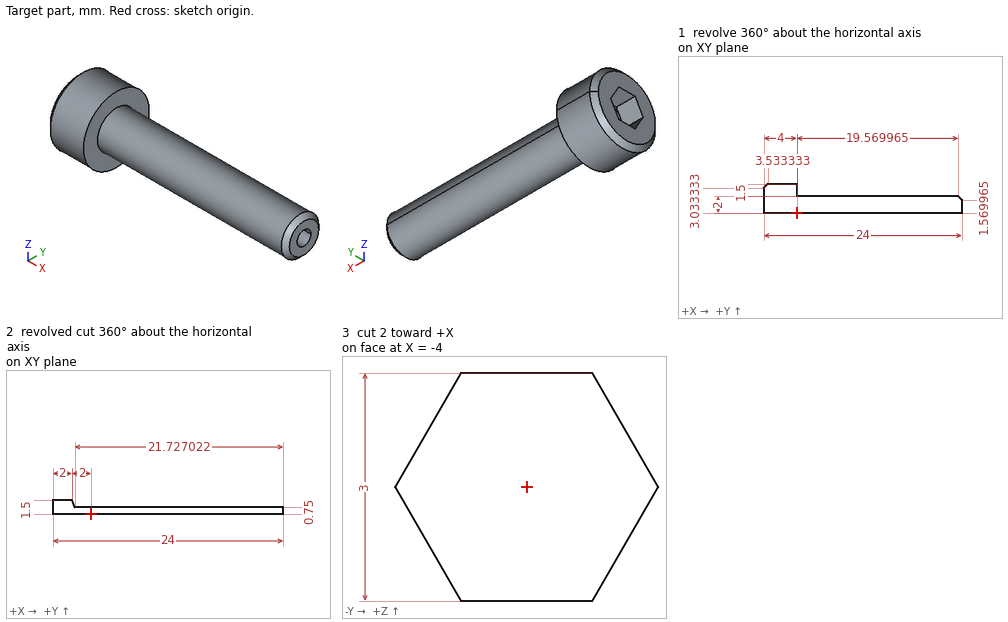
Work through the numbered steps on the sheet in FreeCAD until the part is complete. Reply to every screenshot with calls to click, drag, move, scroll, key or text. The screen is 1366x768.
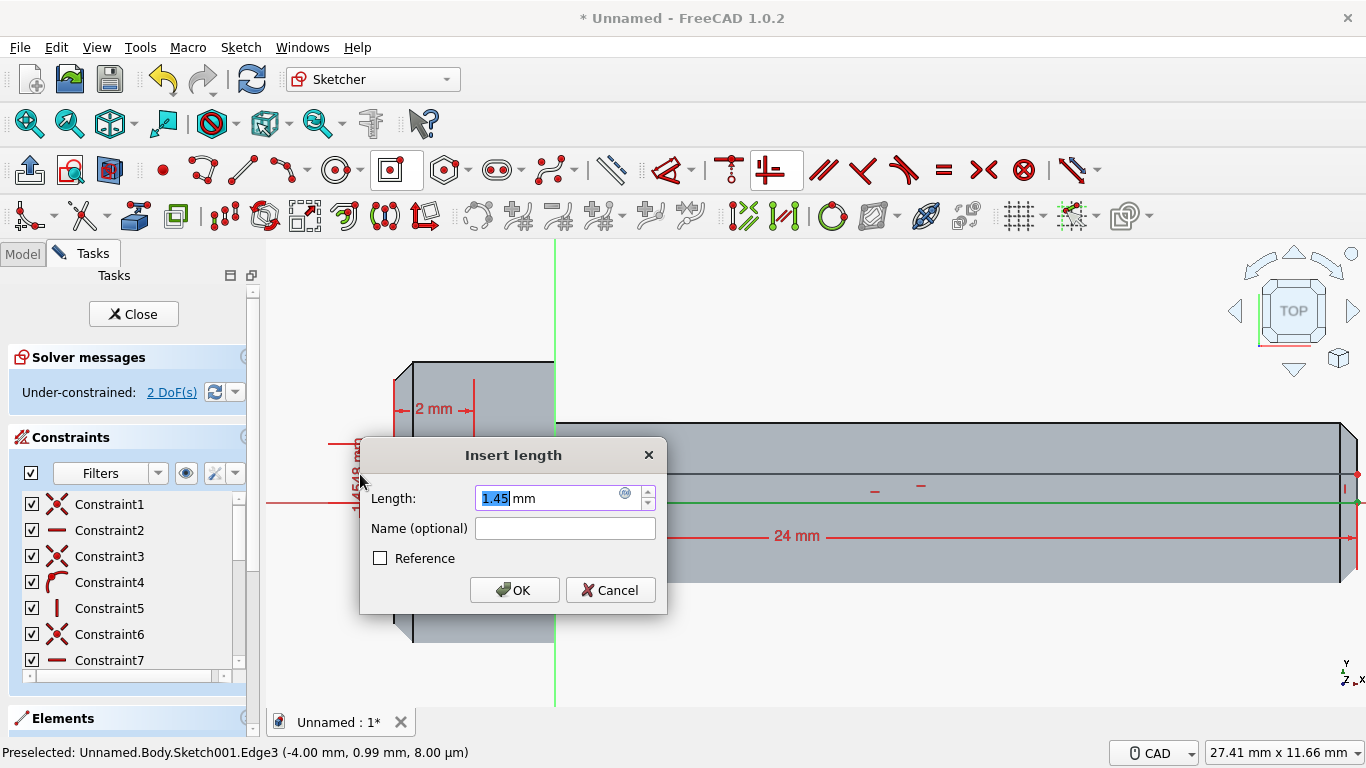
text(1.5)
key(Return)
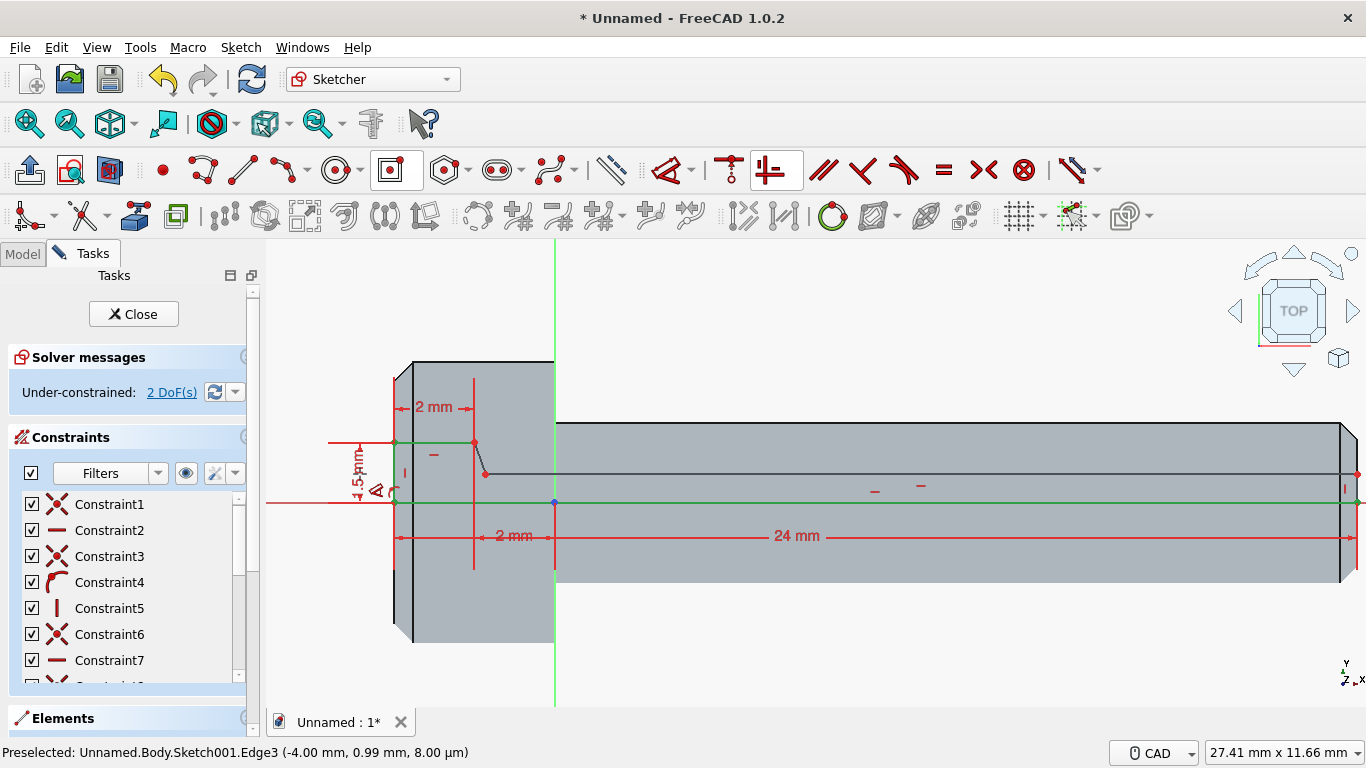
scroll(487, 474, down, 2)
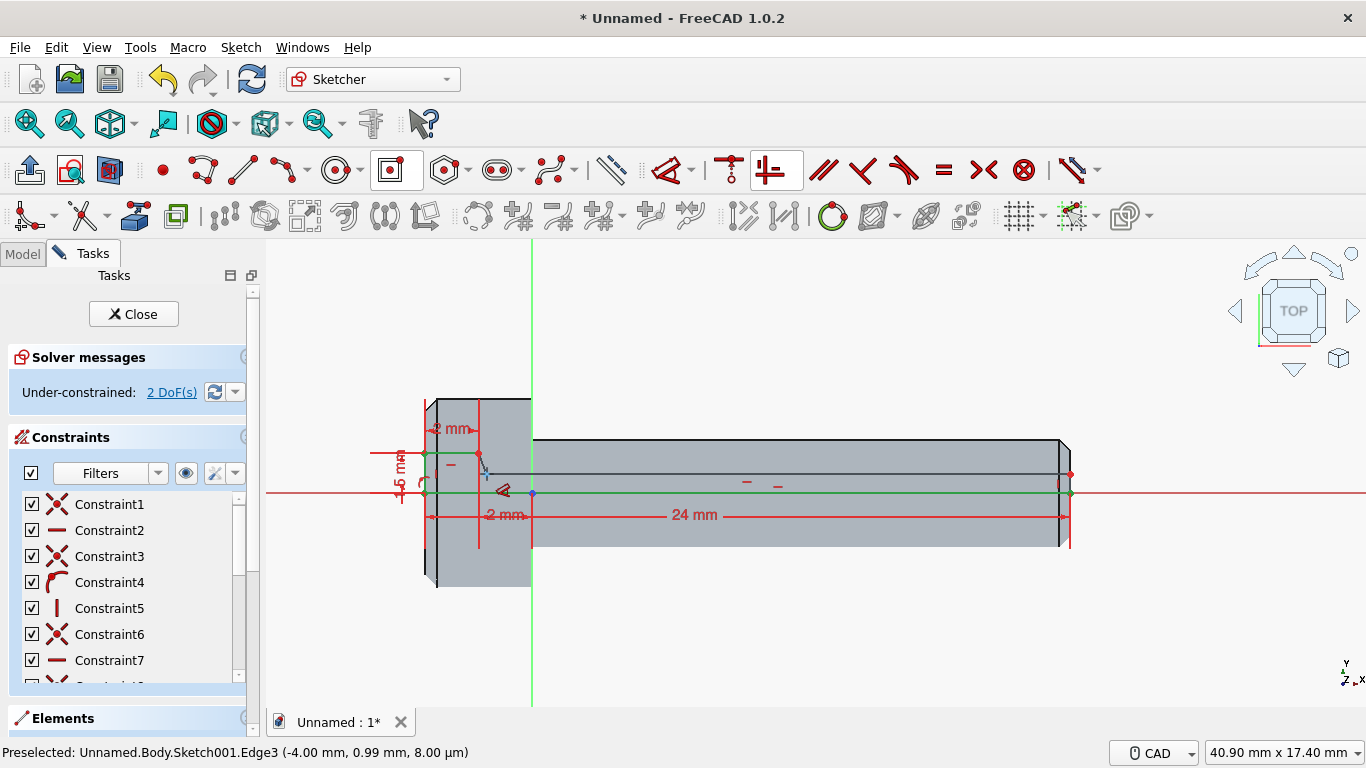
scroll(1070, 486, up, 4)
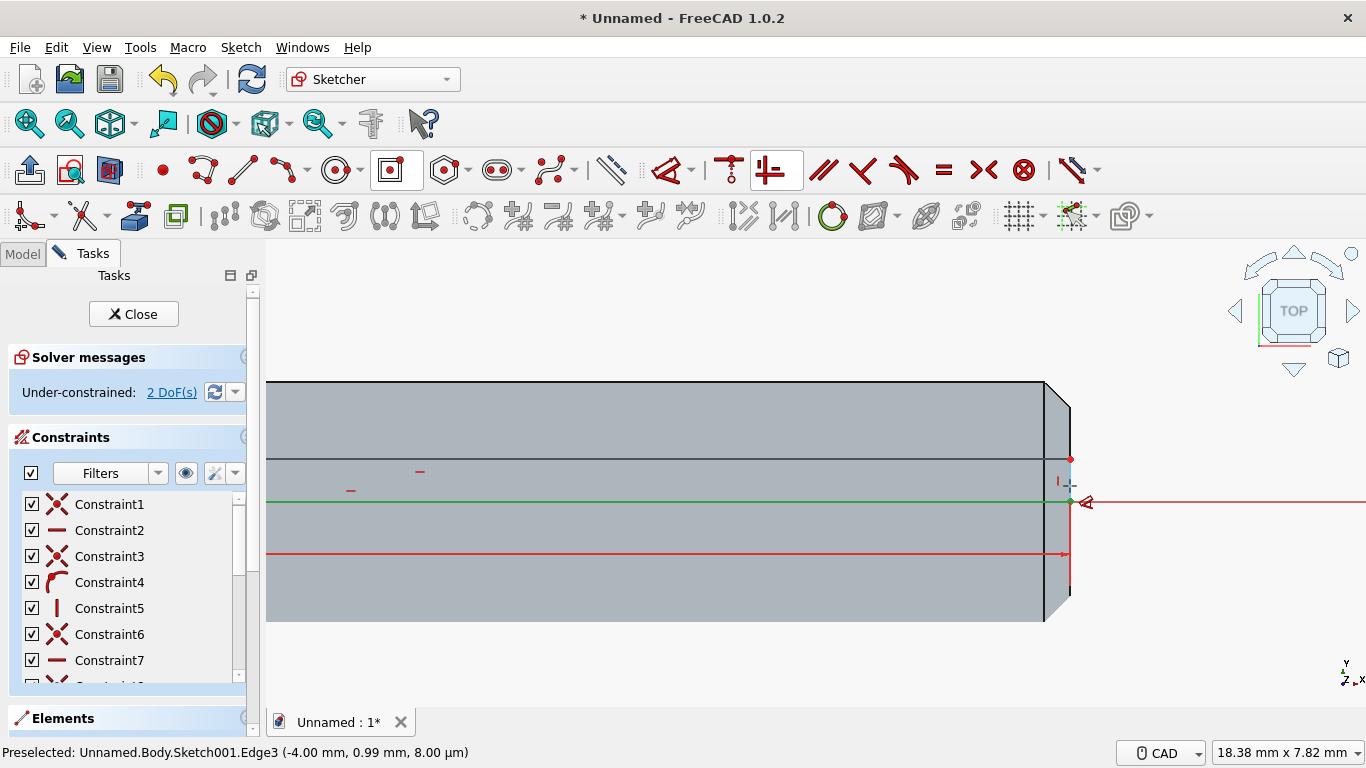
click(1070, 485)
click(1104, 481)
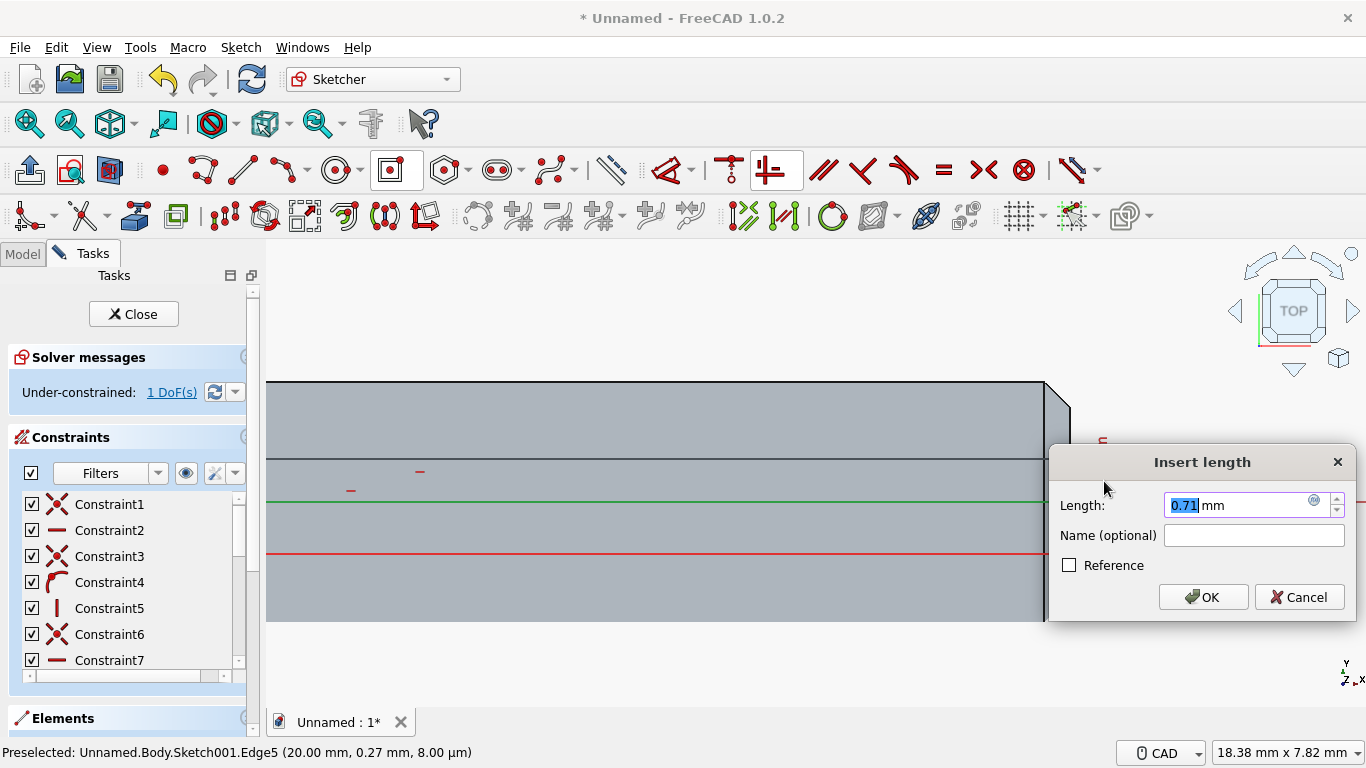
text(0.75)
key(Return)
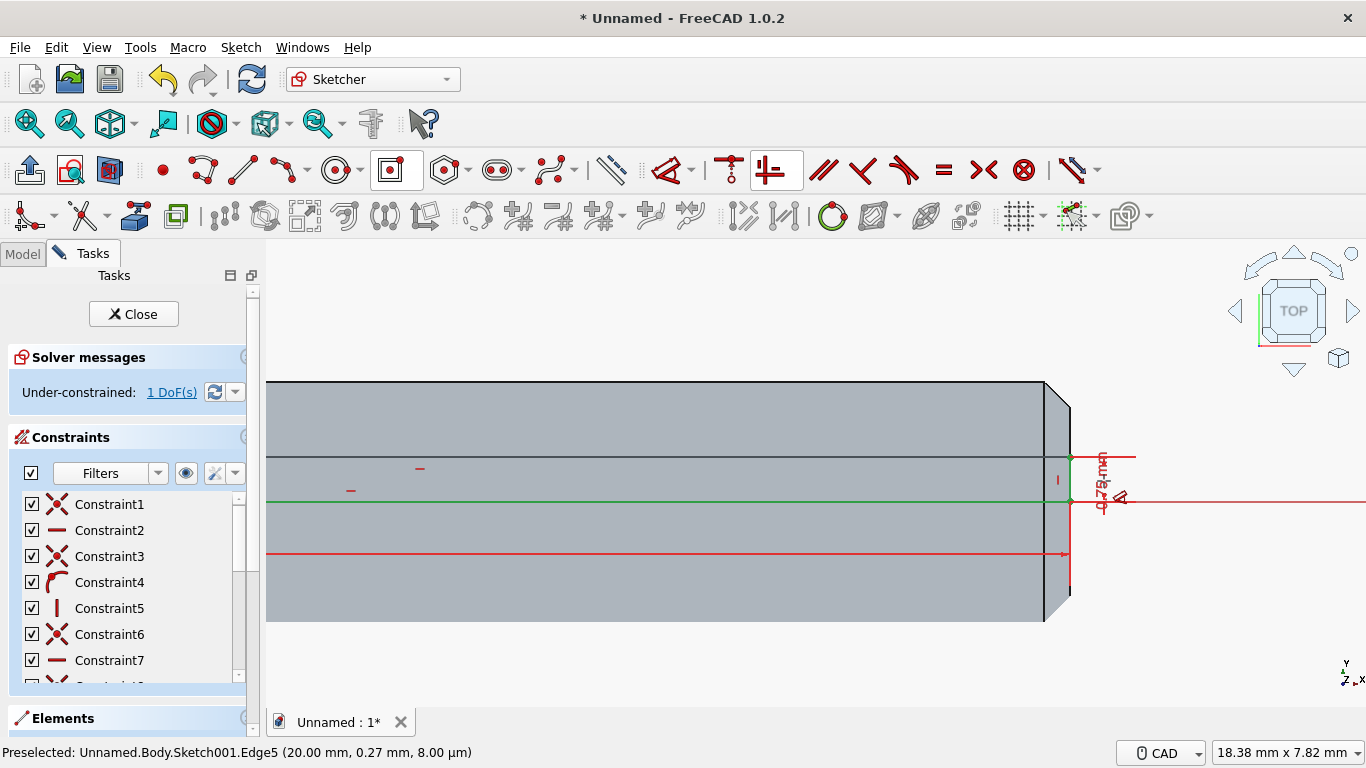
click(680, 457)
click(682, 423)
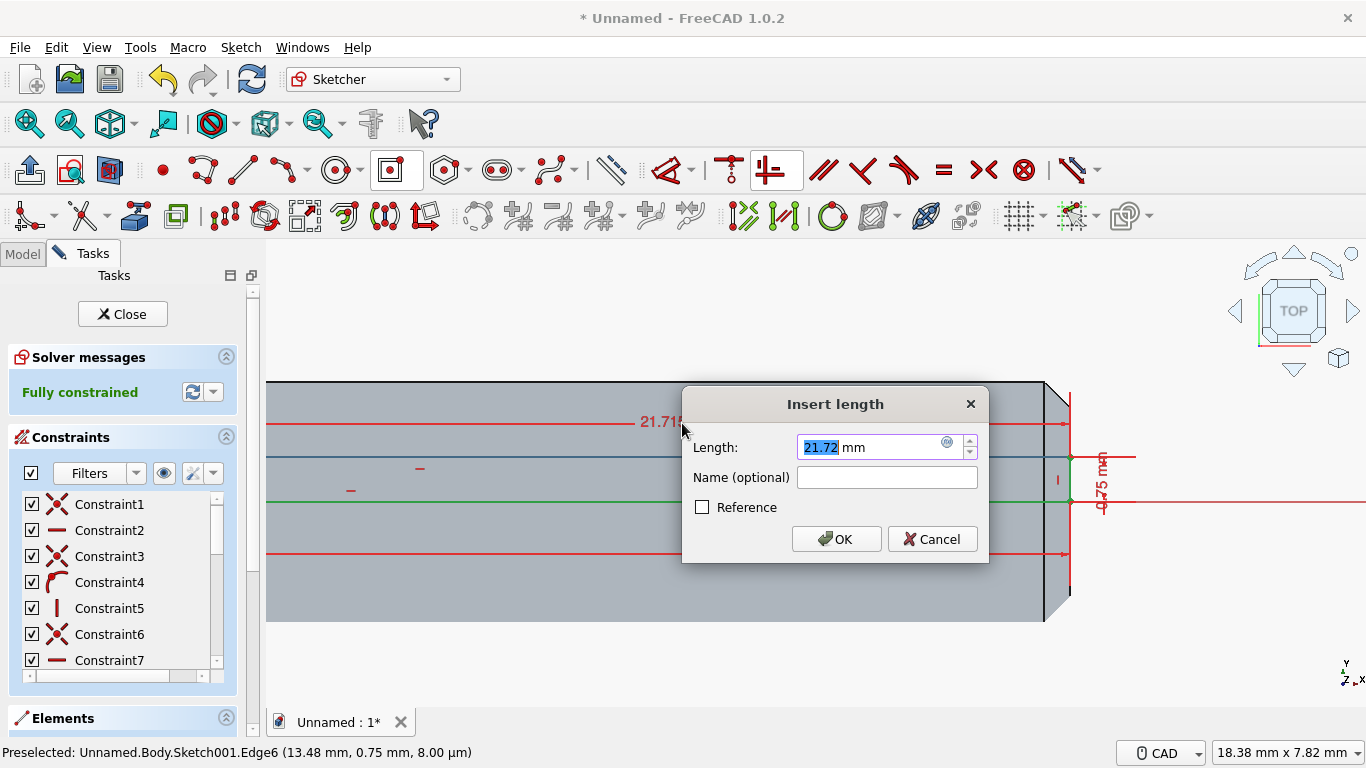
text(21.727022)
key(Return)
key(Escape)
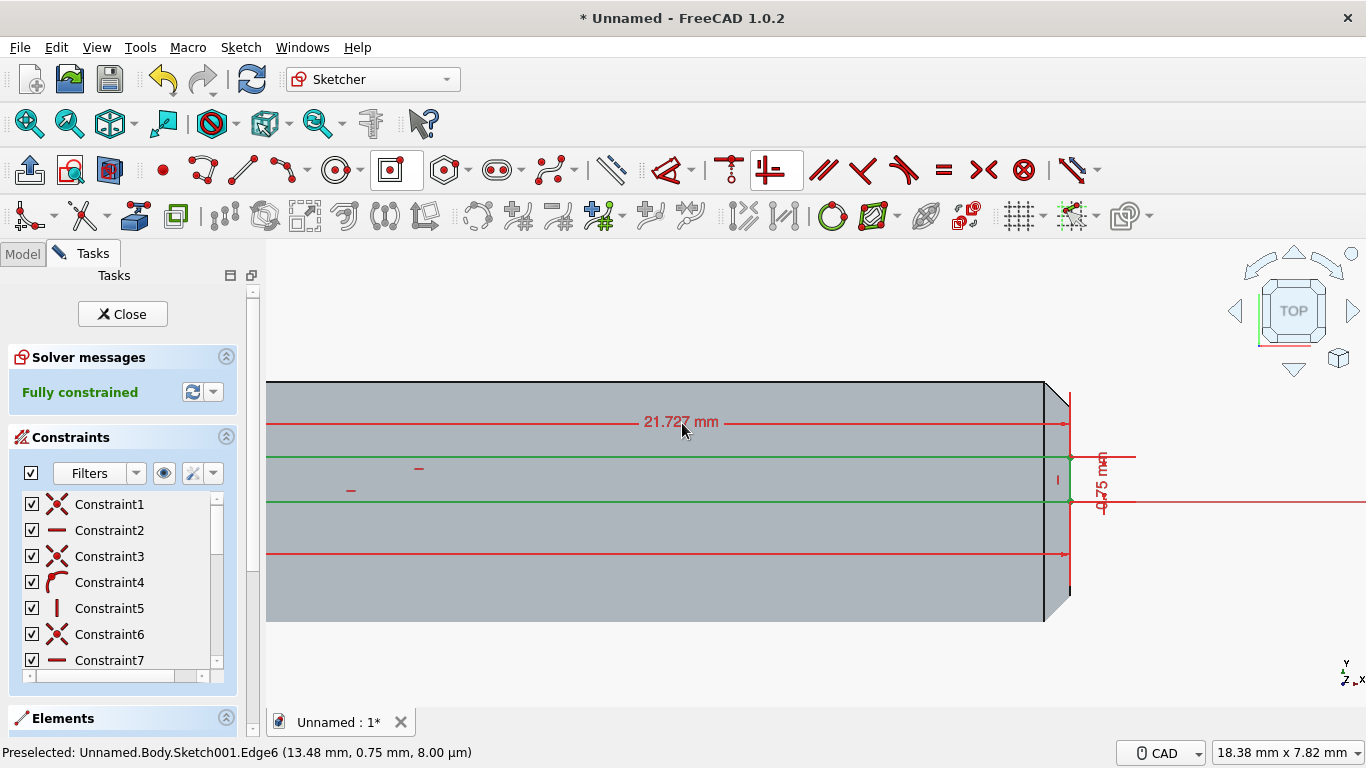
click(123, 314)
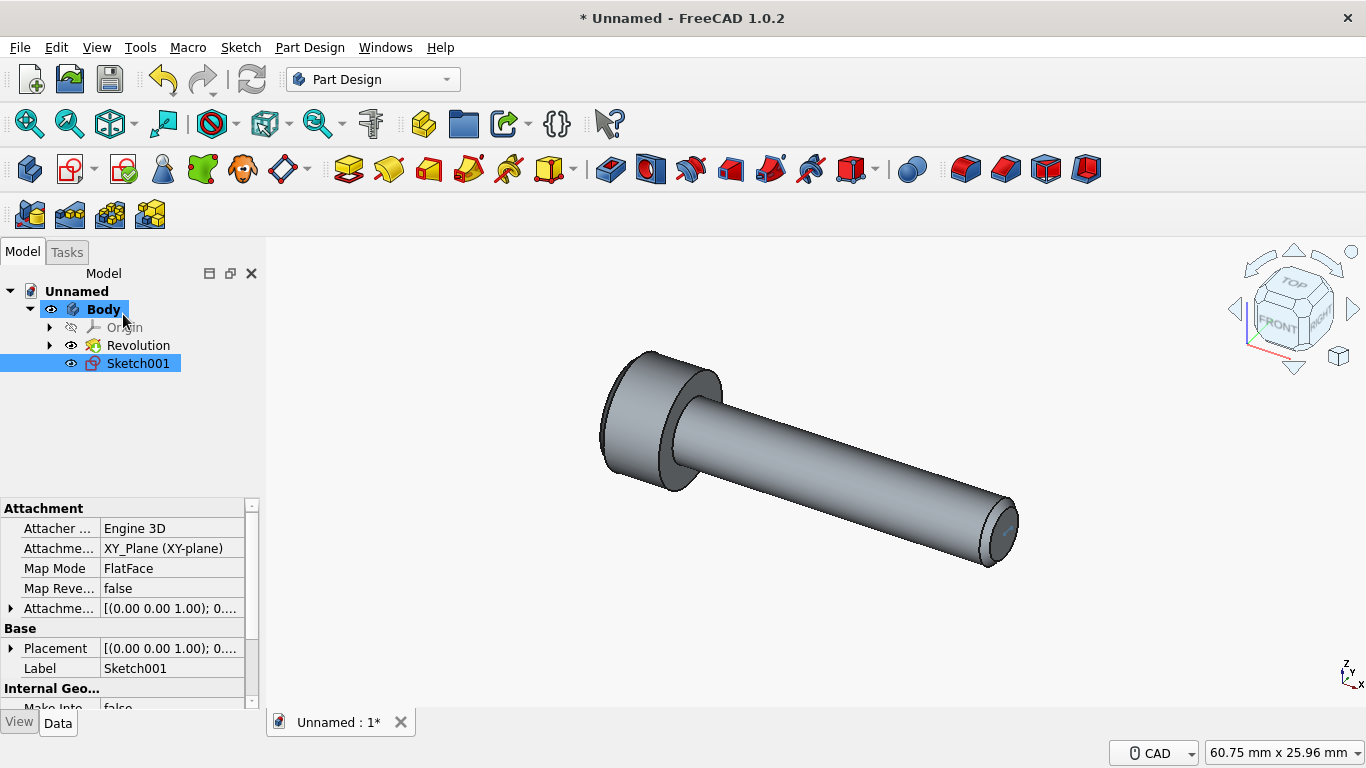
click(692, 170)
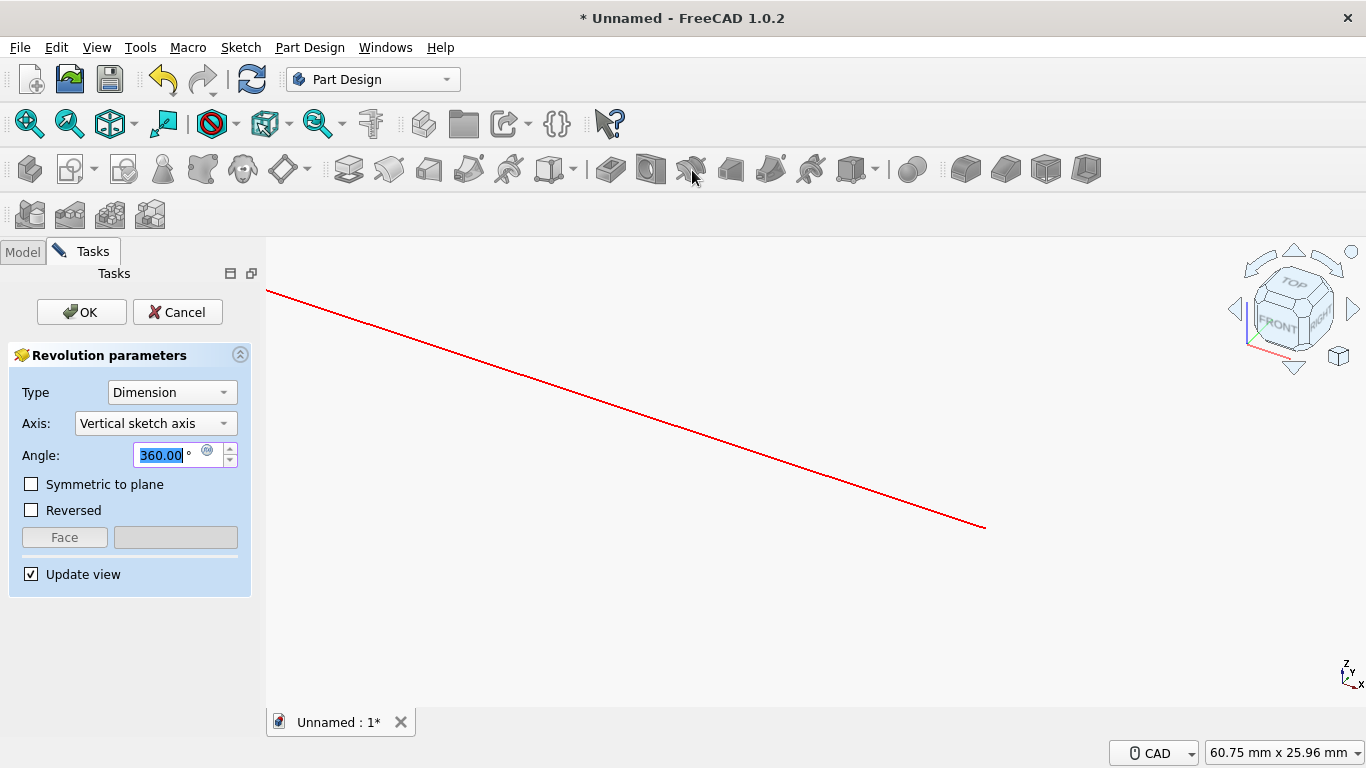
click(156, 424)